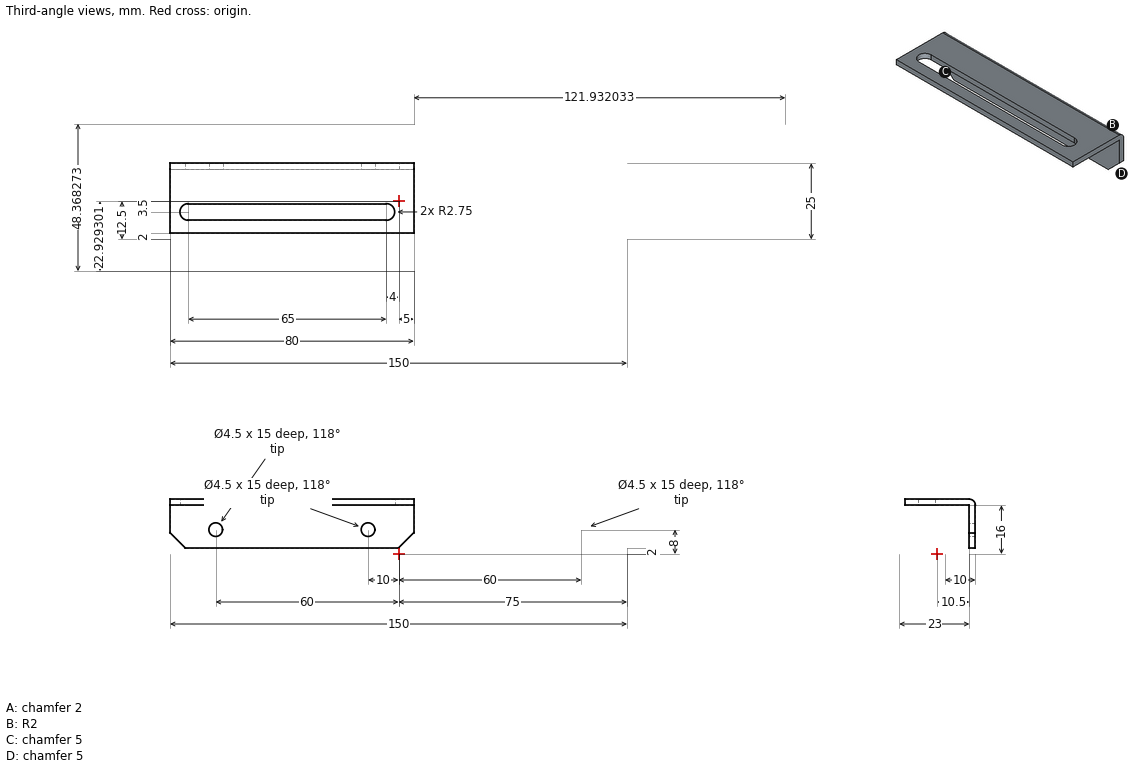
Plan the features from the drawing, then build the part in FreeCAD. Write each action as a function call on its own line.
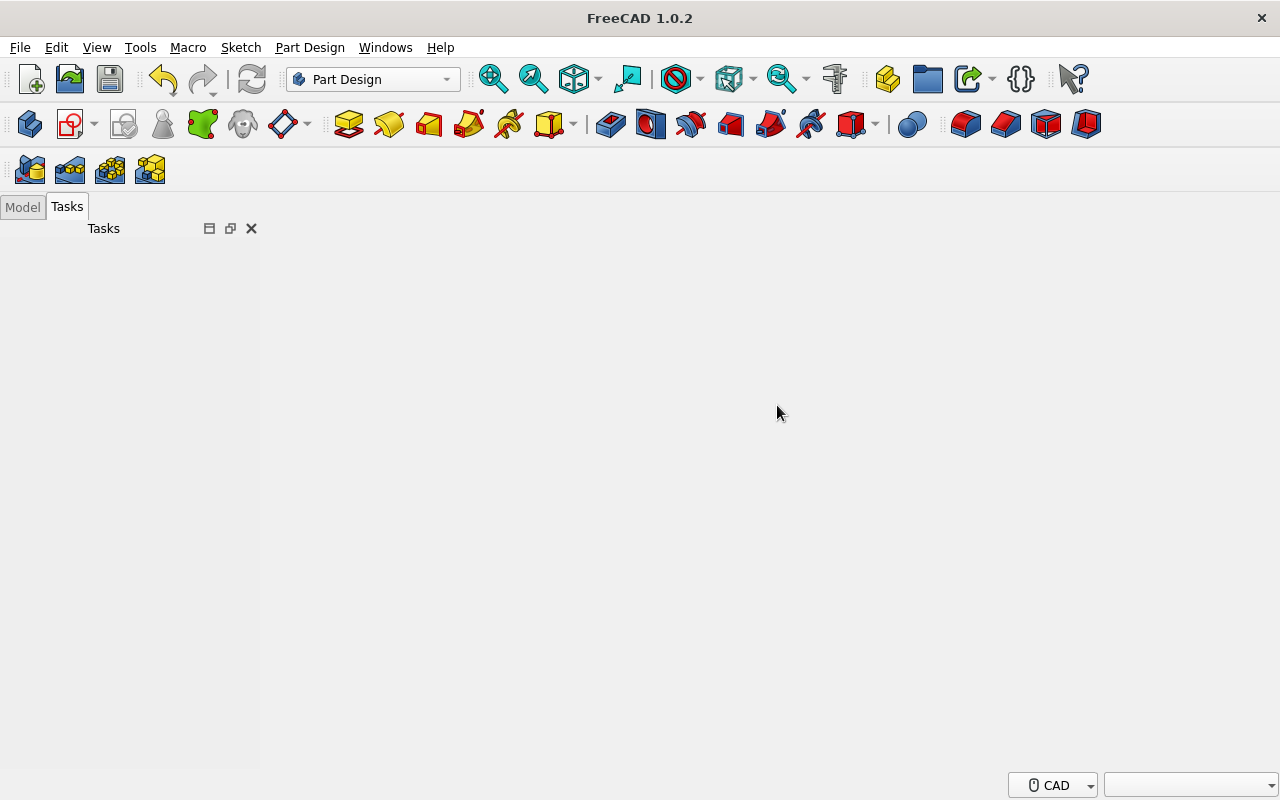
click(30, 80)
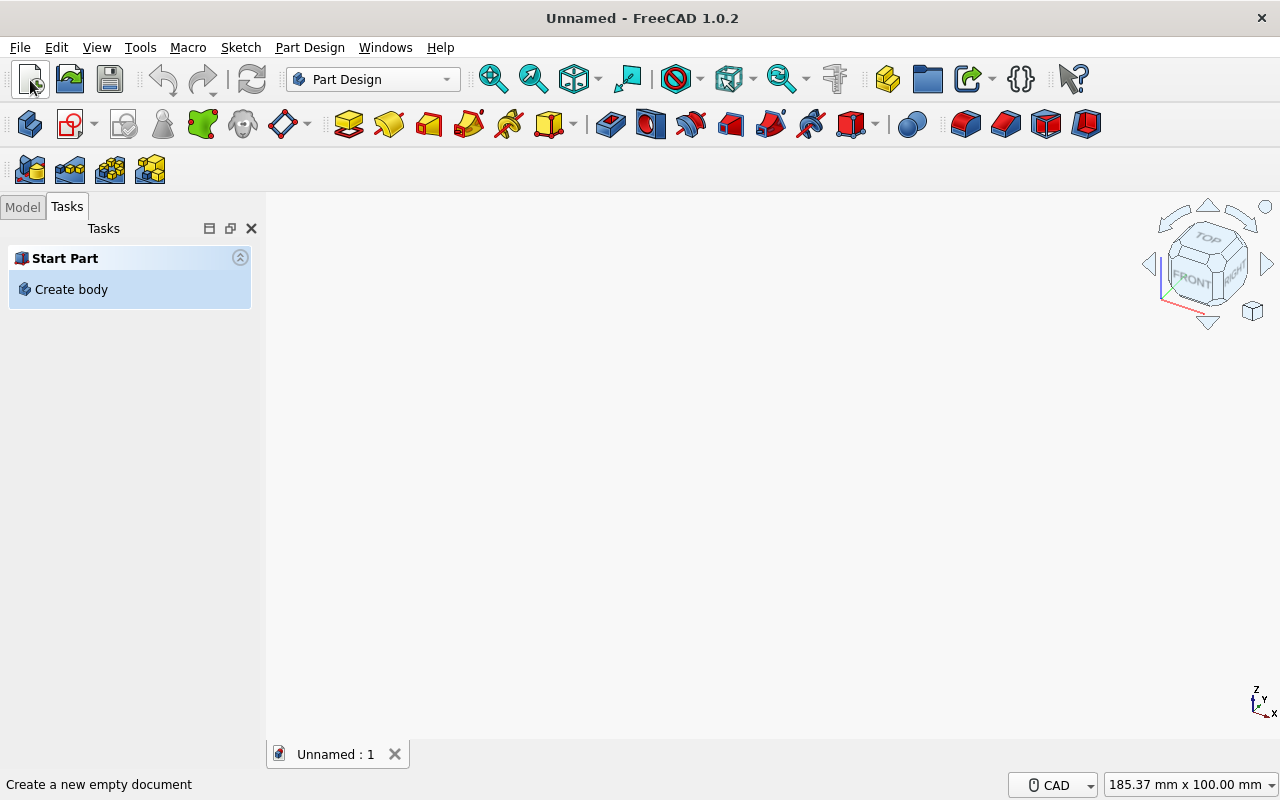
click(70, 124)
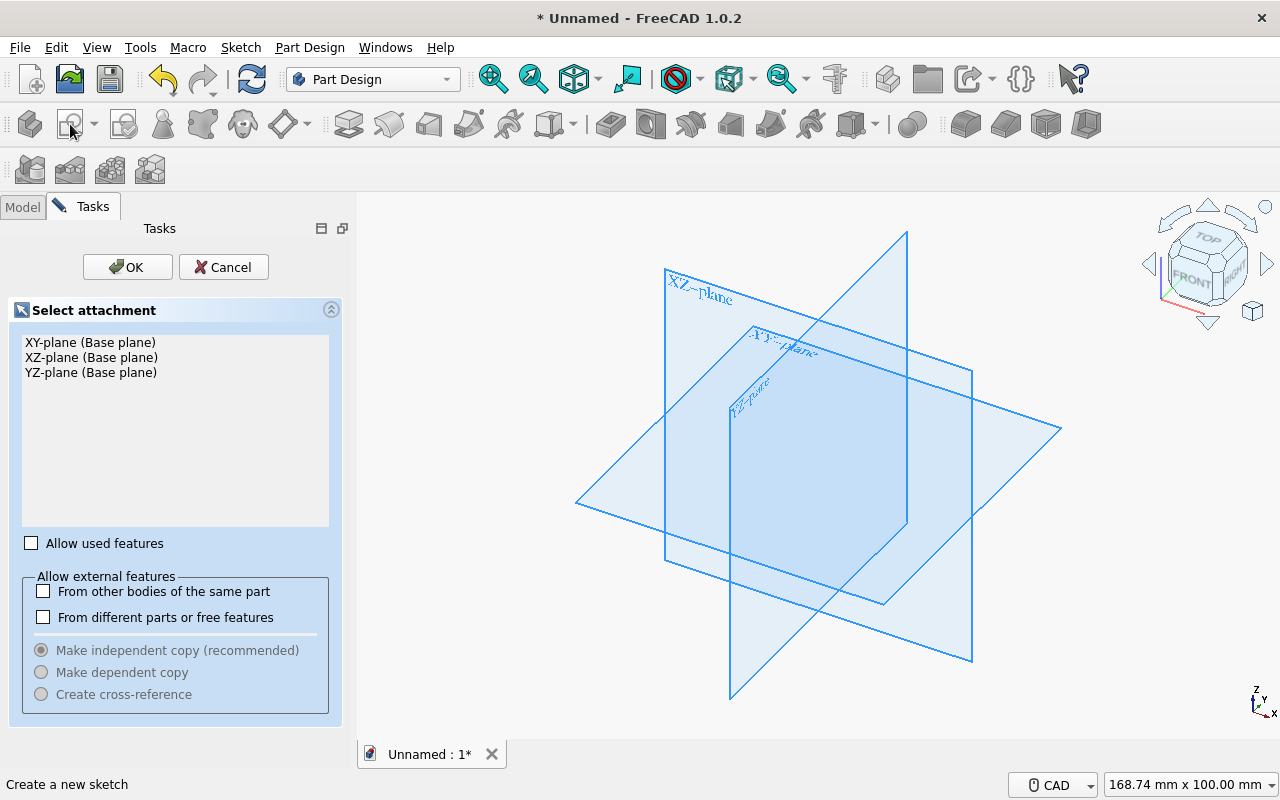
click(82, 342)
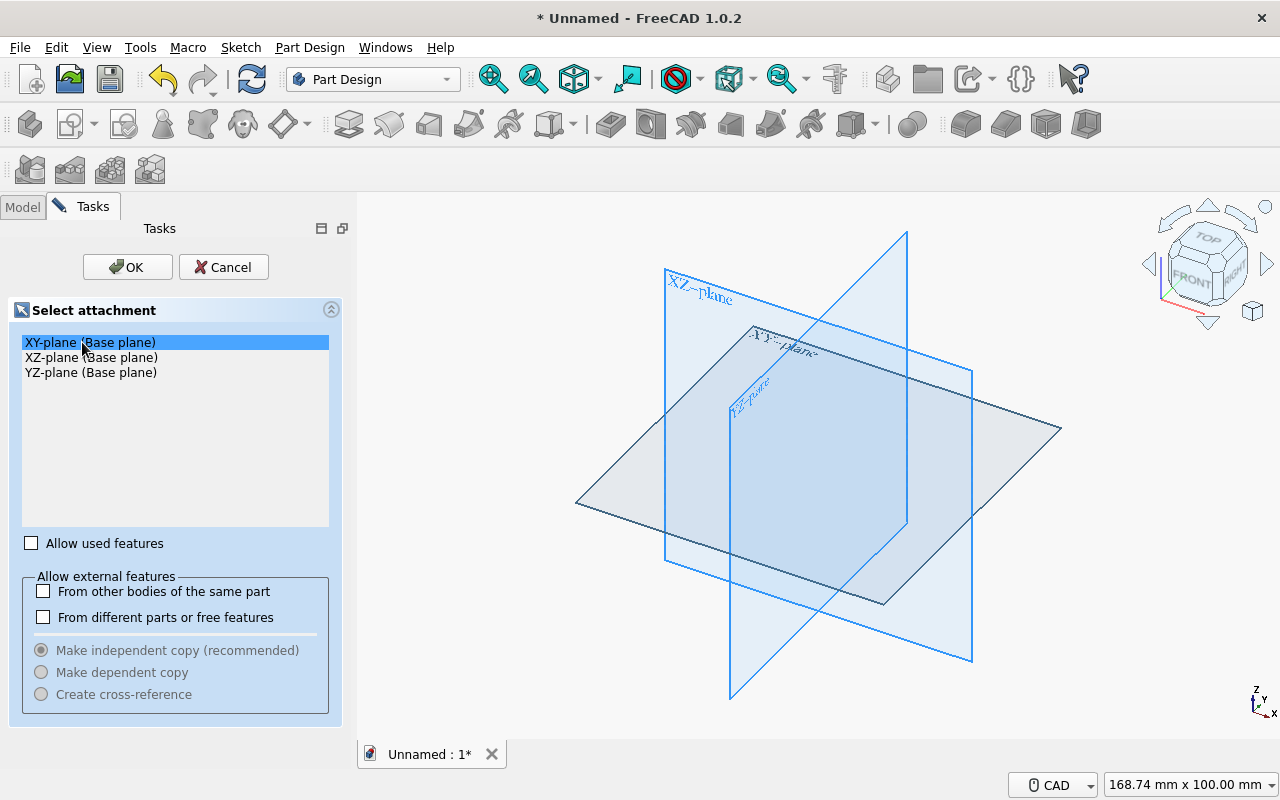
click(128, 267)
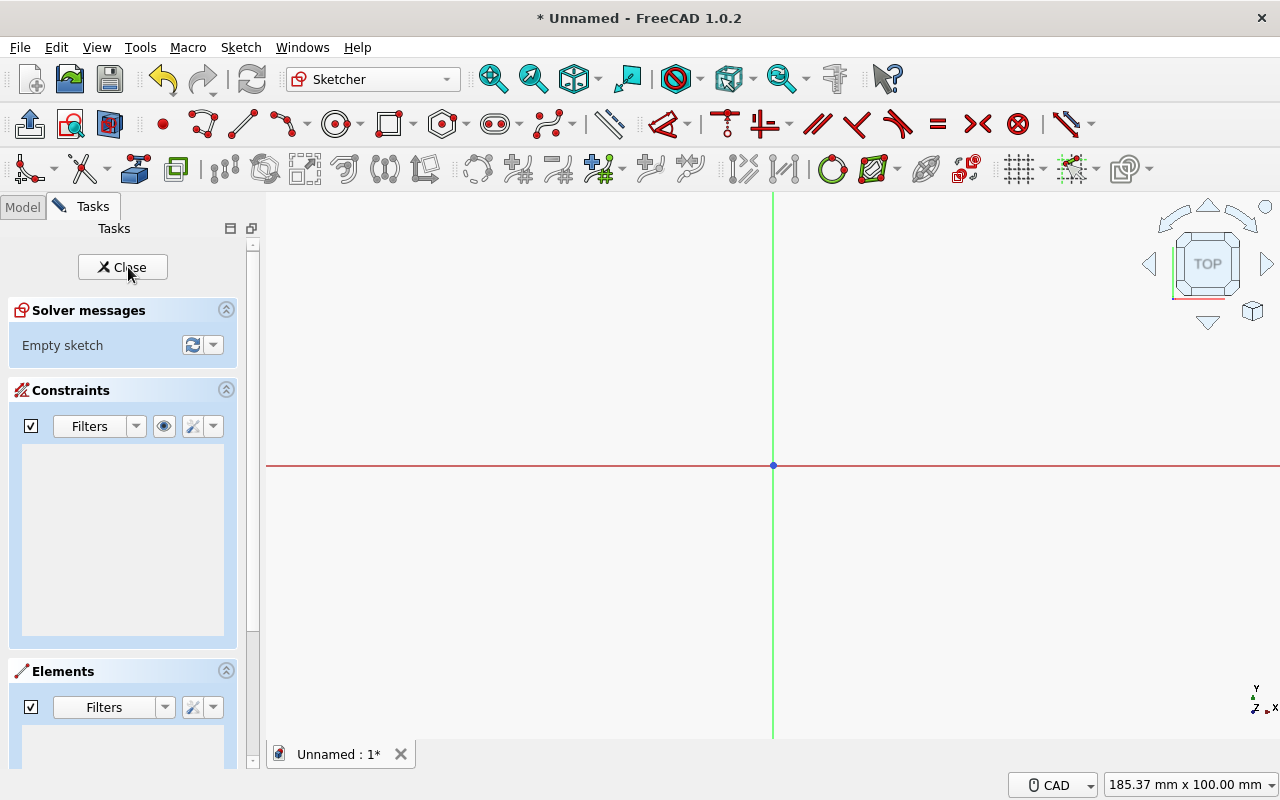
scroll(565, 466, down, 2)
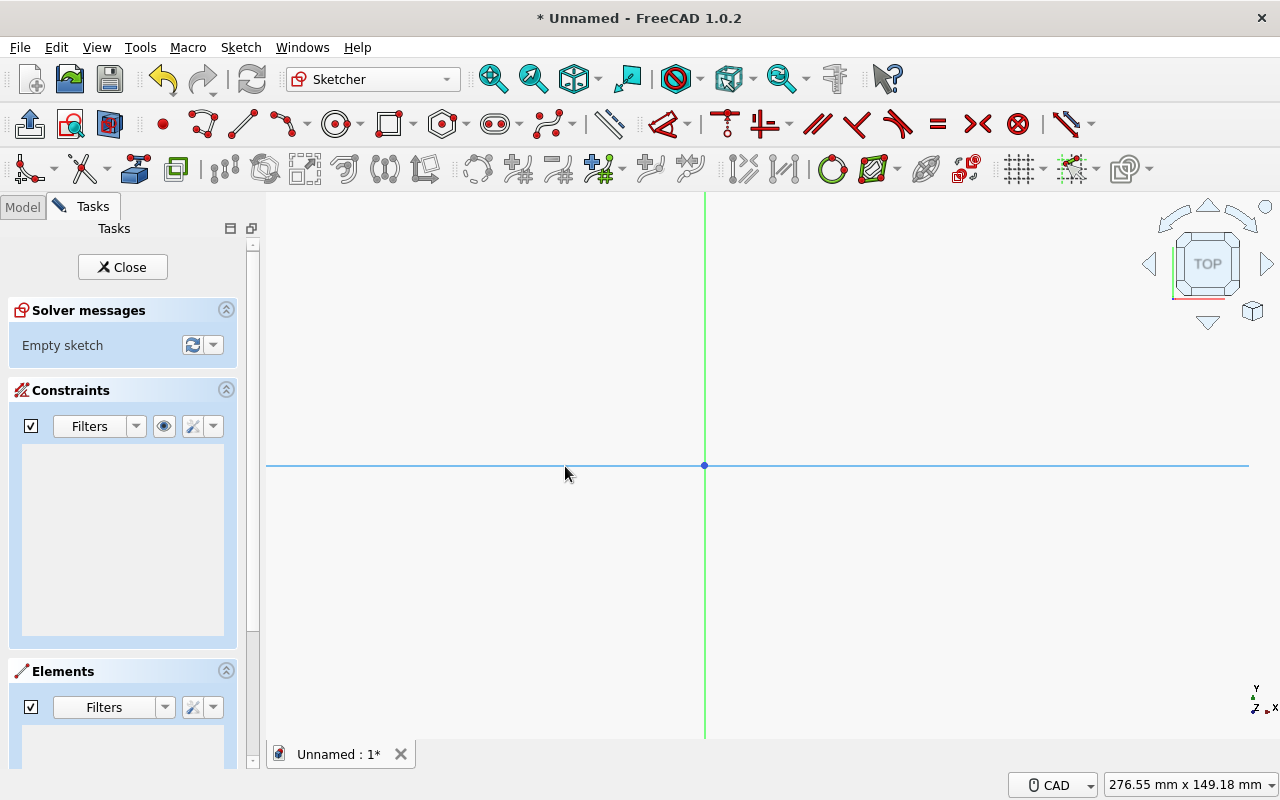
click(416, 124)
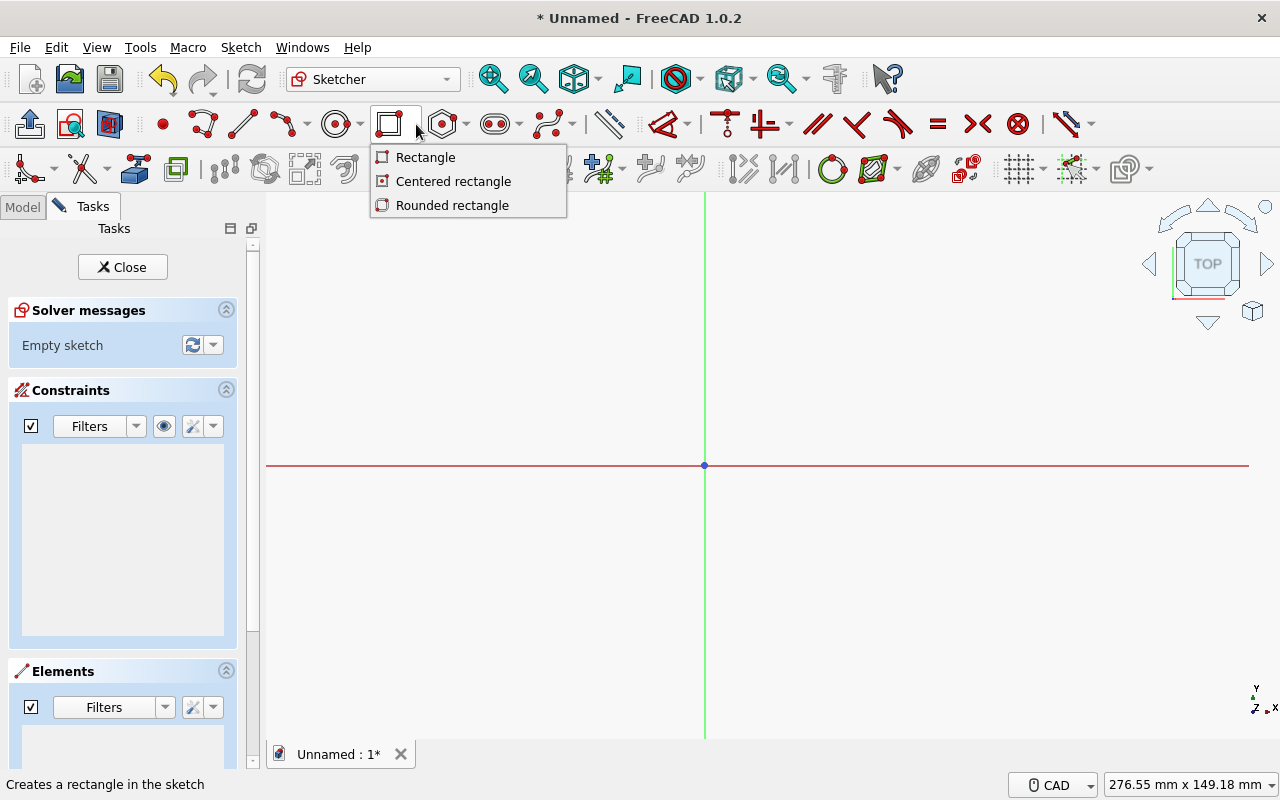
click(468, 181)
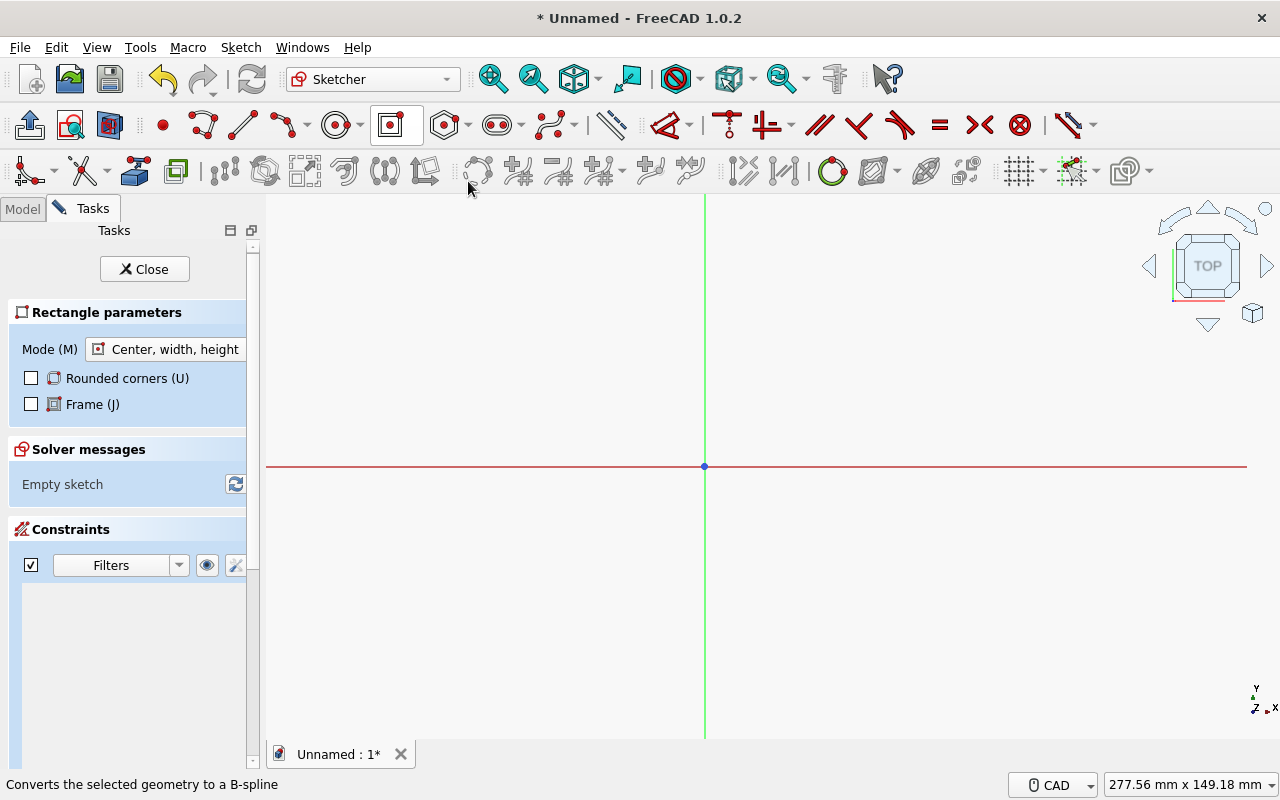
click(705, 467)
click(979, 421)
key(Escape)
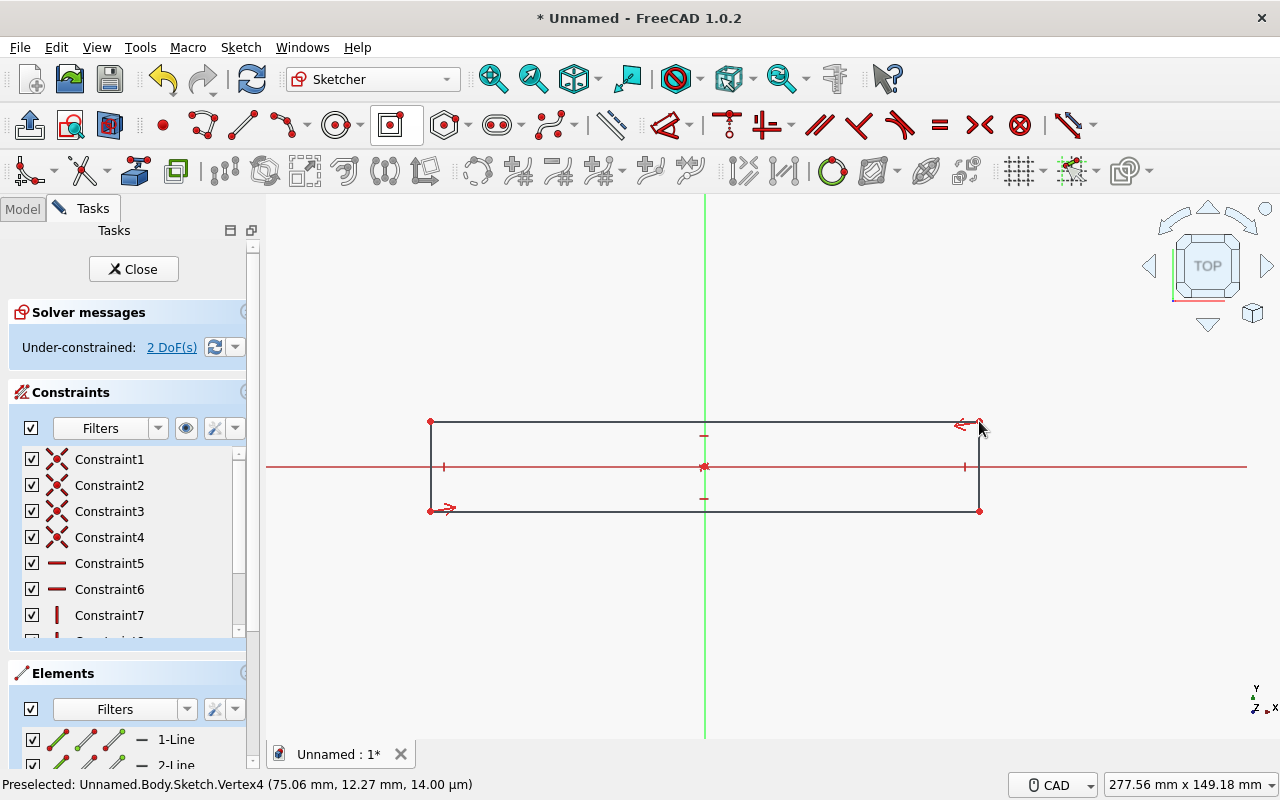
click(666, 126)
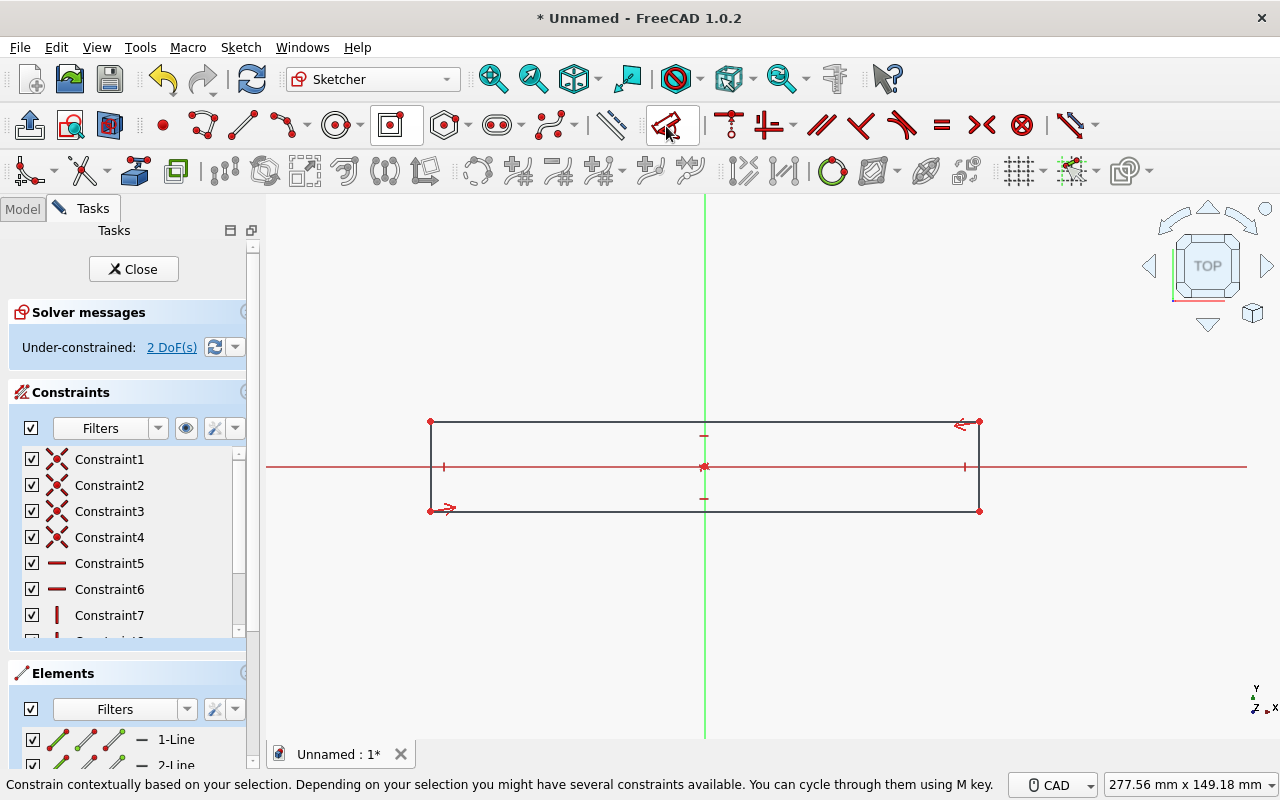
click(979, 485)
click(1013, 446)